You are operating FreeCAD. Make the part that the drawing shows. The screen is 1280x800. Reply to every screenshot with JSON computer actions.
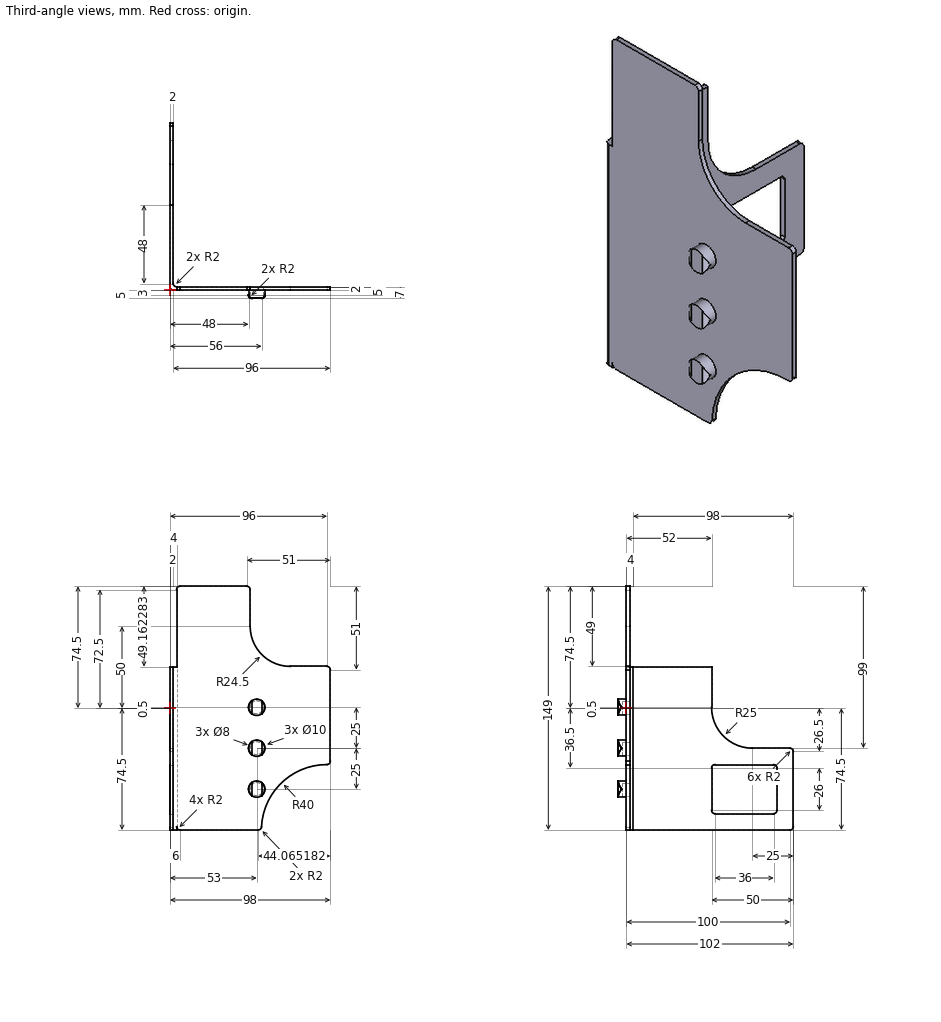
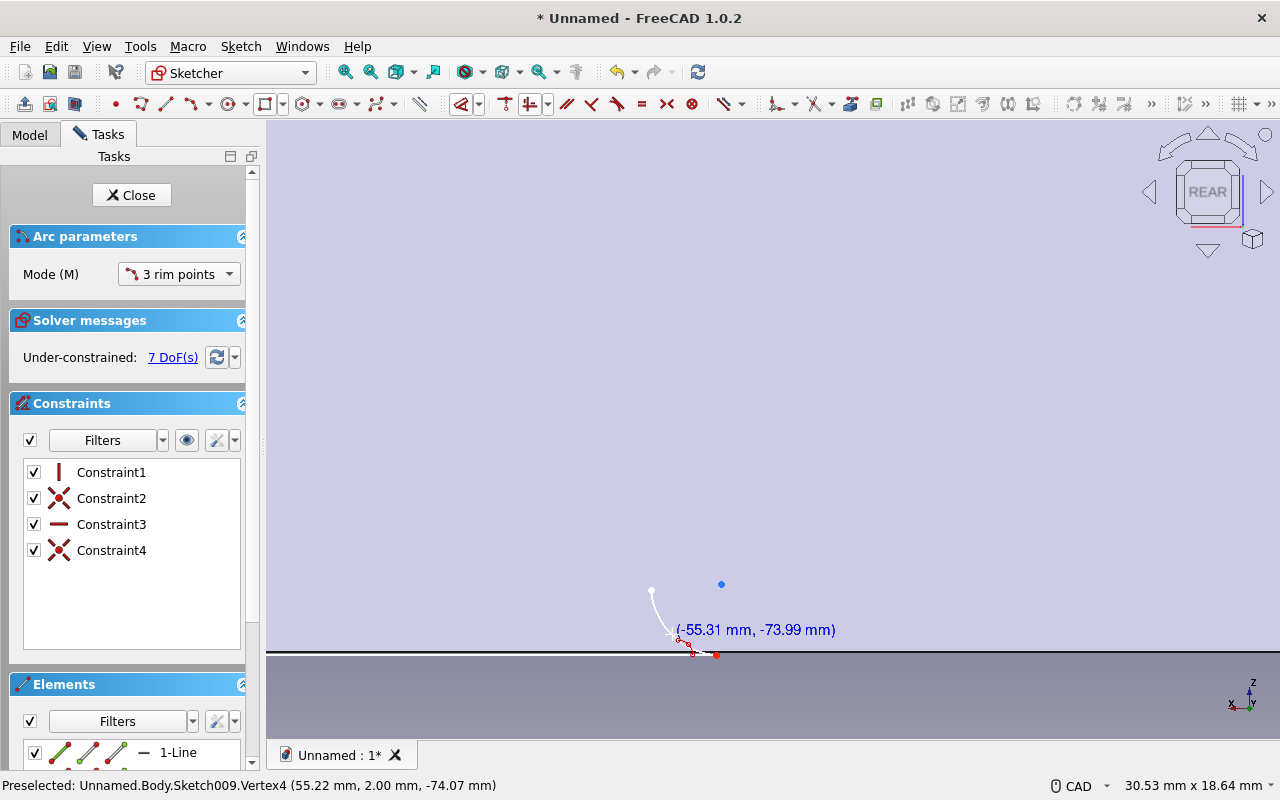
{"action": "scroll", "coordinate": [669, 630], "scroll_direction": "down", "scroll_amount": 9}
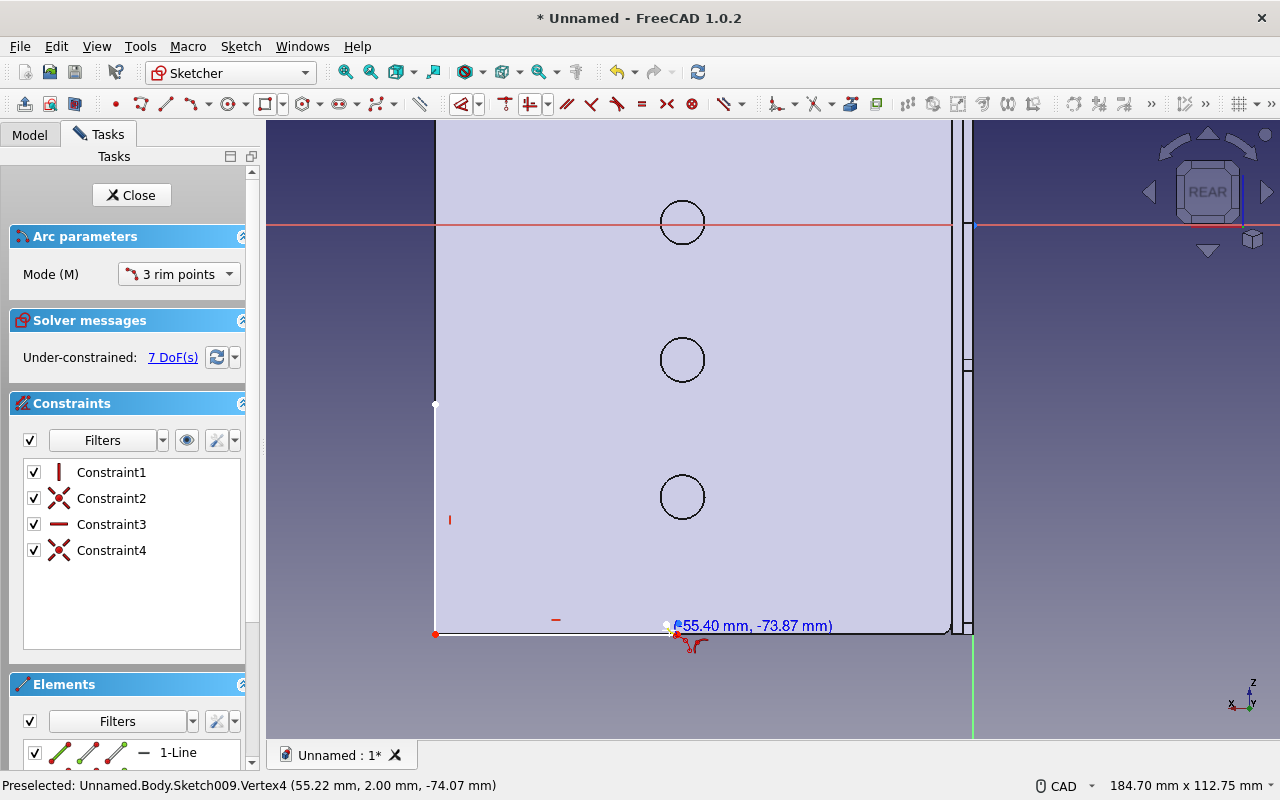
{"action": "scroll", "coordinate": [666, 624], "scroll_direction": "up", "scroll_amount": 3}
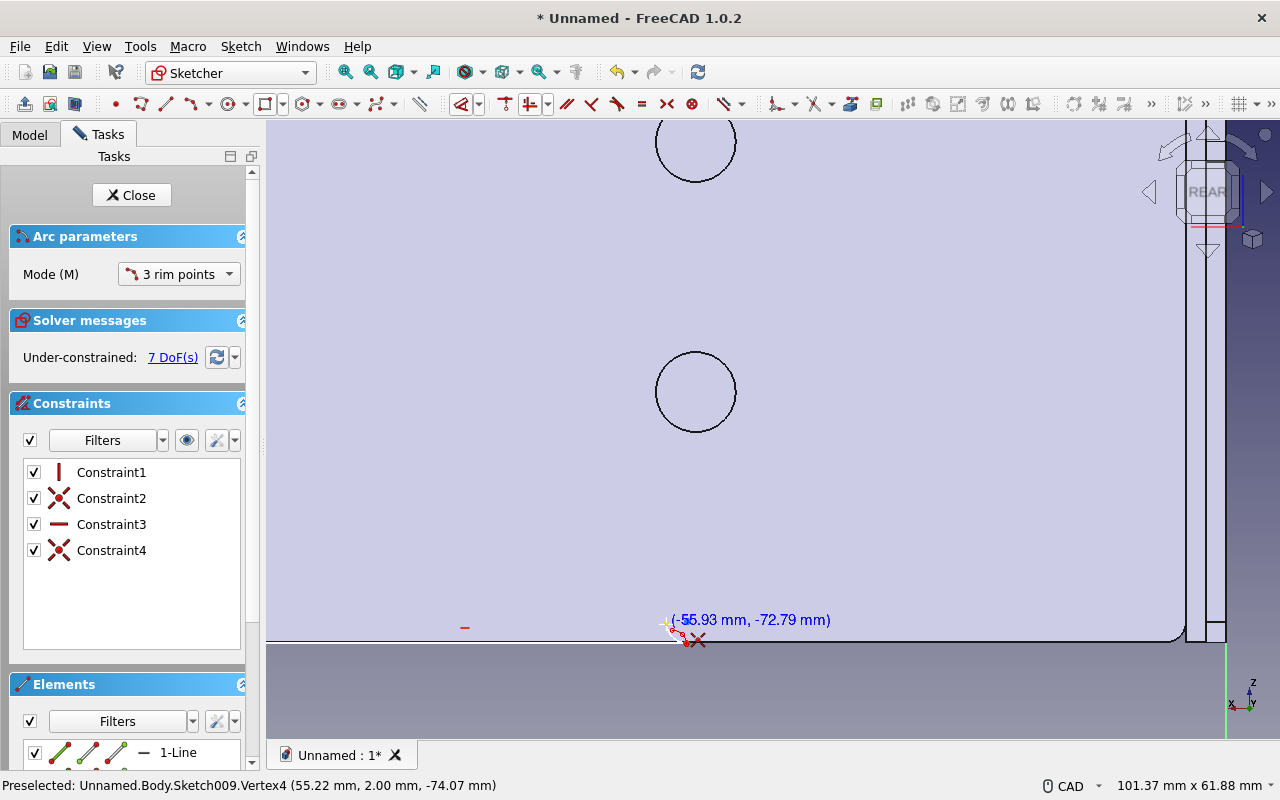
{"action": "left_click", "coordinate": [666, 624]}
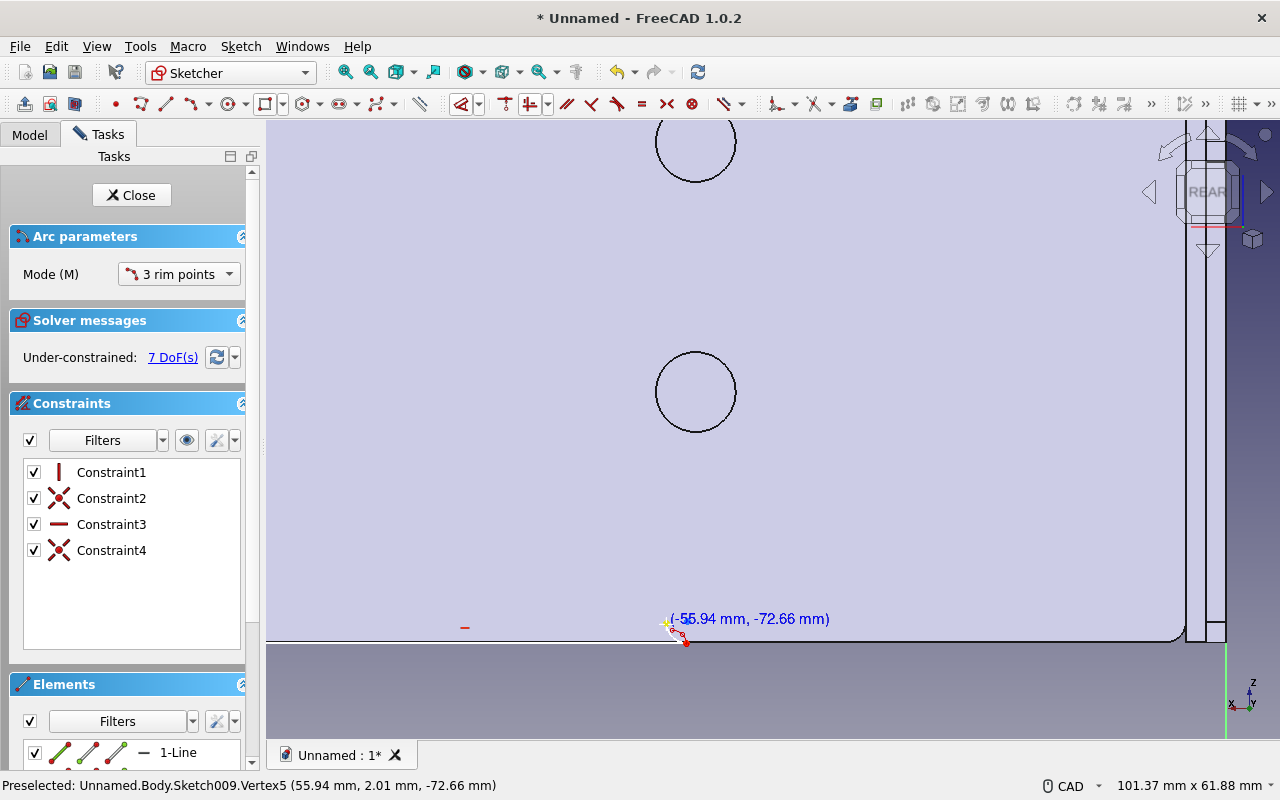
{"action": "scroll", "coordinate": [666, 624], "scroll_direction": "down", "scroll_amount": 3}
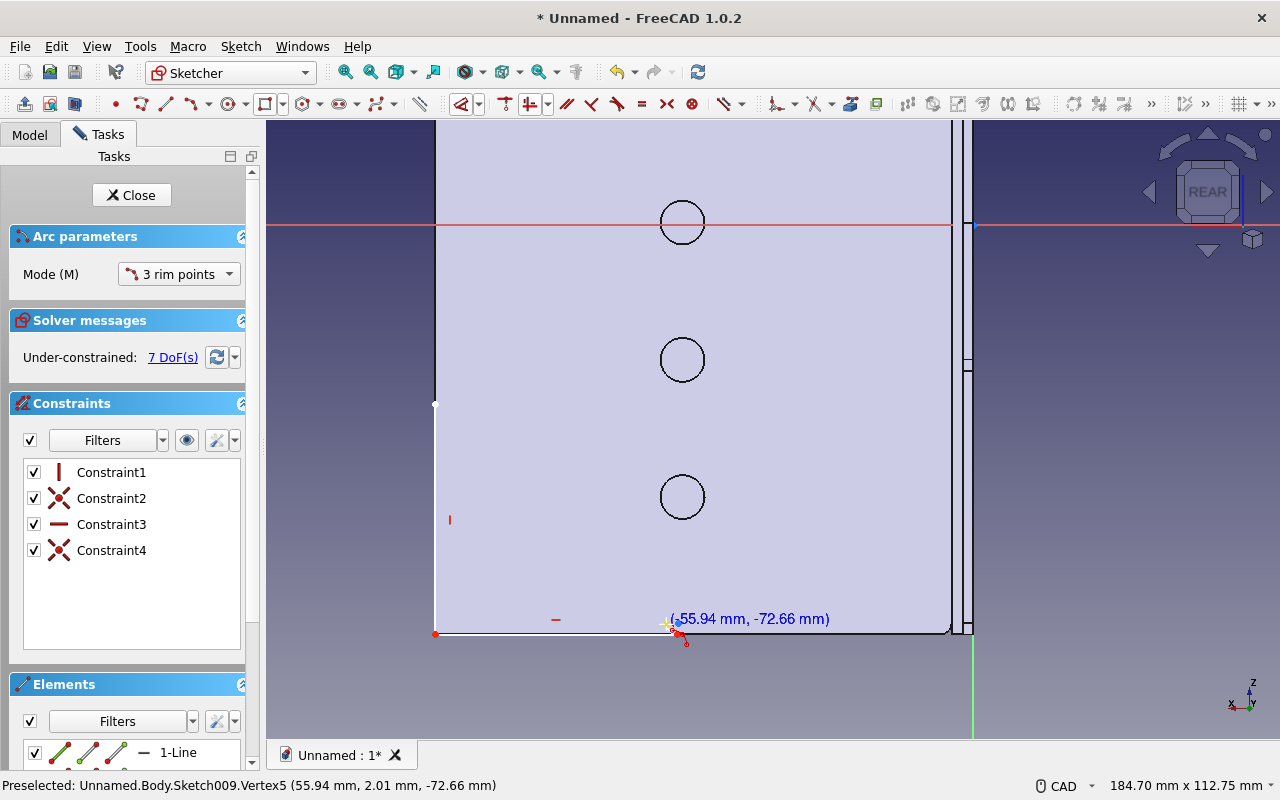
{"action": "scroll", "coordinate": [446, 415], "scroll_direction": "up", "scroll_amount": 2}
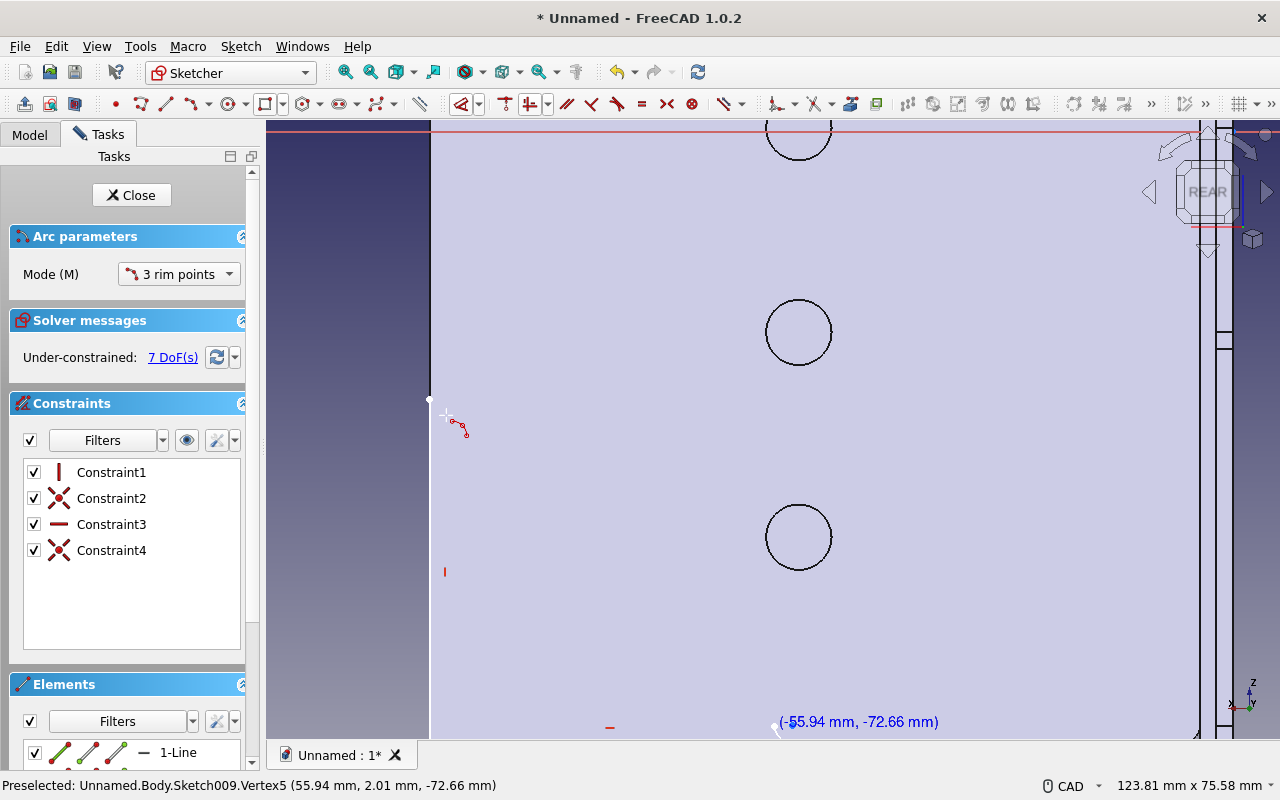
{"action": "left_click", "coordinate": [447, 414]}
{"action": "left_click", "coordinate": [673, 505]}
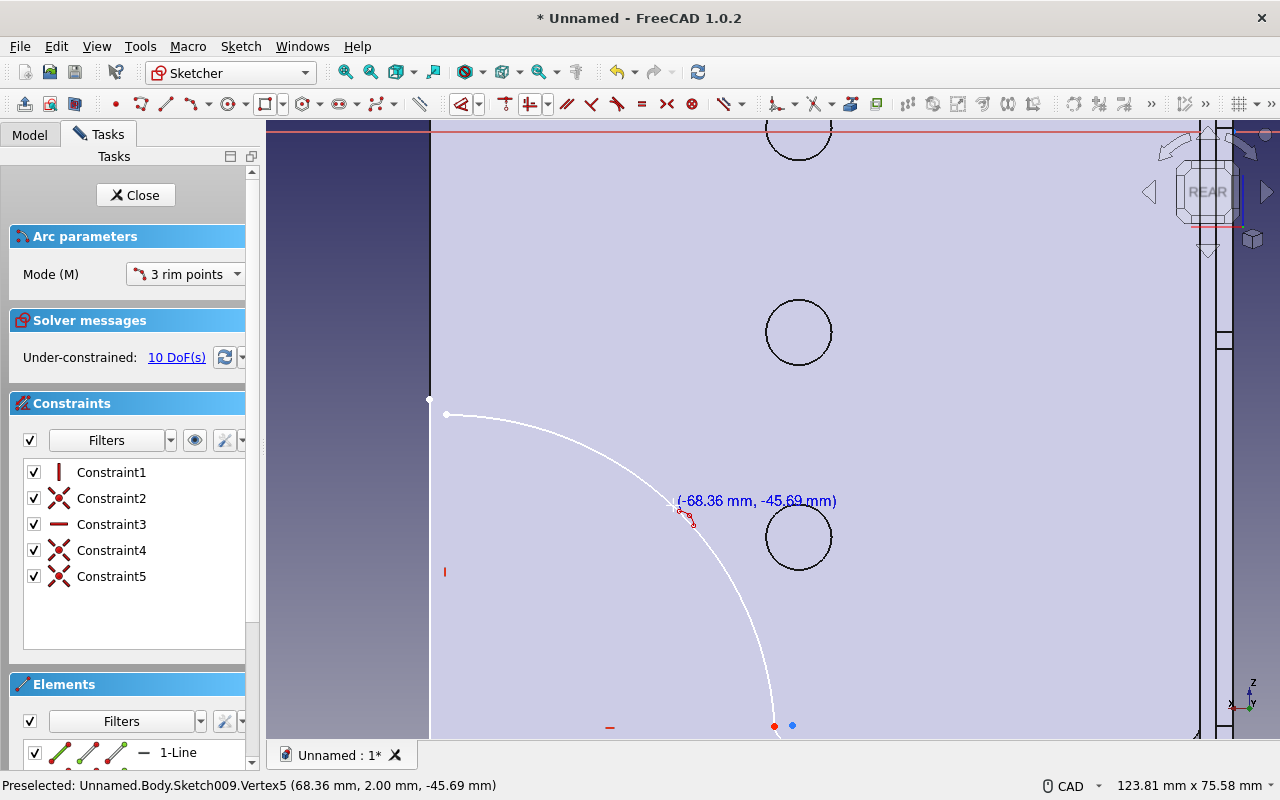
{"action": "left_click", "coordinate": [447, 415]}
{"action": "left_click", "coordinate": [430, 400]}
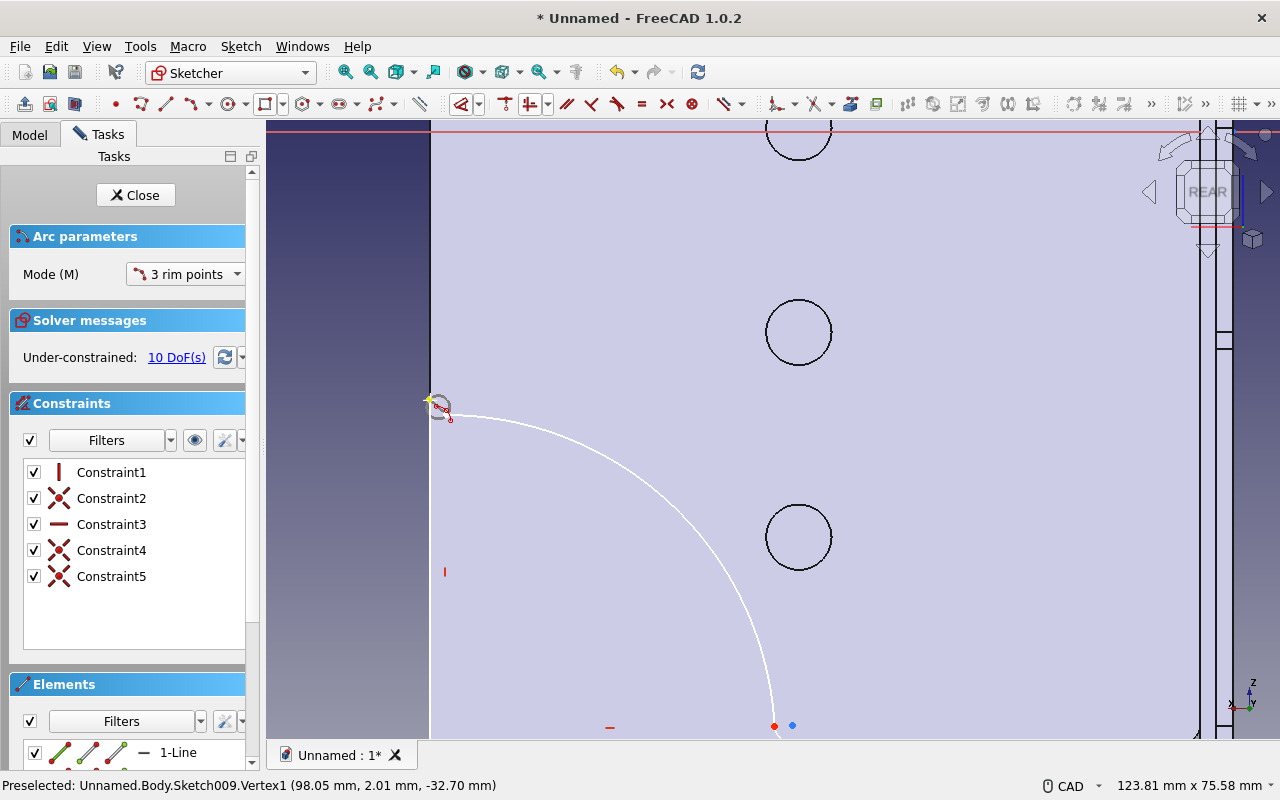
{"action": "scroll", "coordinate": [435, 410], "scroll_direction": "up", "scroll_amount": 6}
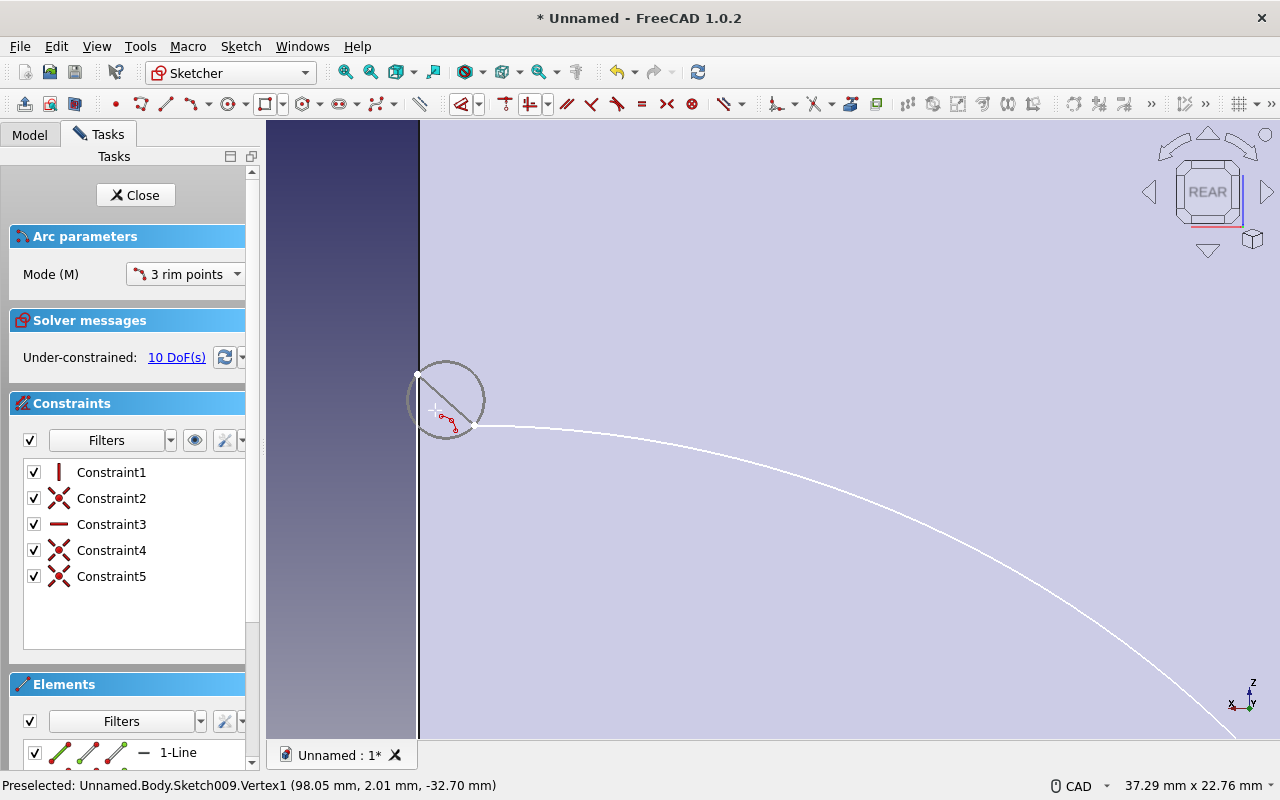
{"action": "left_click", "coordinate": [435, 407]}
{"action": "key", "text": "Escape"}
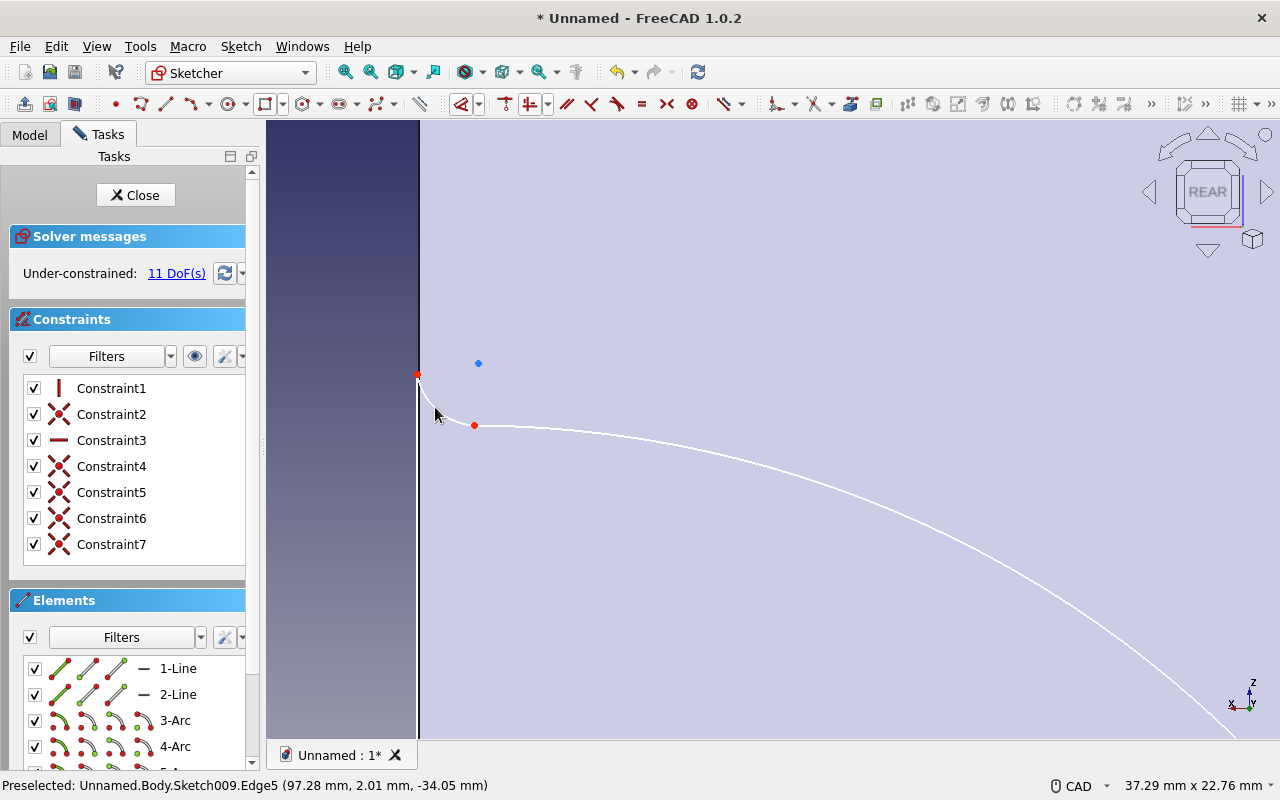
{"action": "scroll", "coordinate": [440, 412], "scroll_direction": "down", "scroll_amount": 8}